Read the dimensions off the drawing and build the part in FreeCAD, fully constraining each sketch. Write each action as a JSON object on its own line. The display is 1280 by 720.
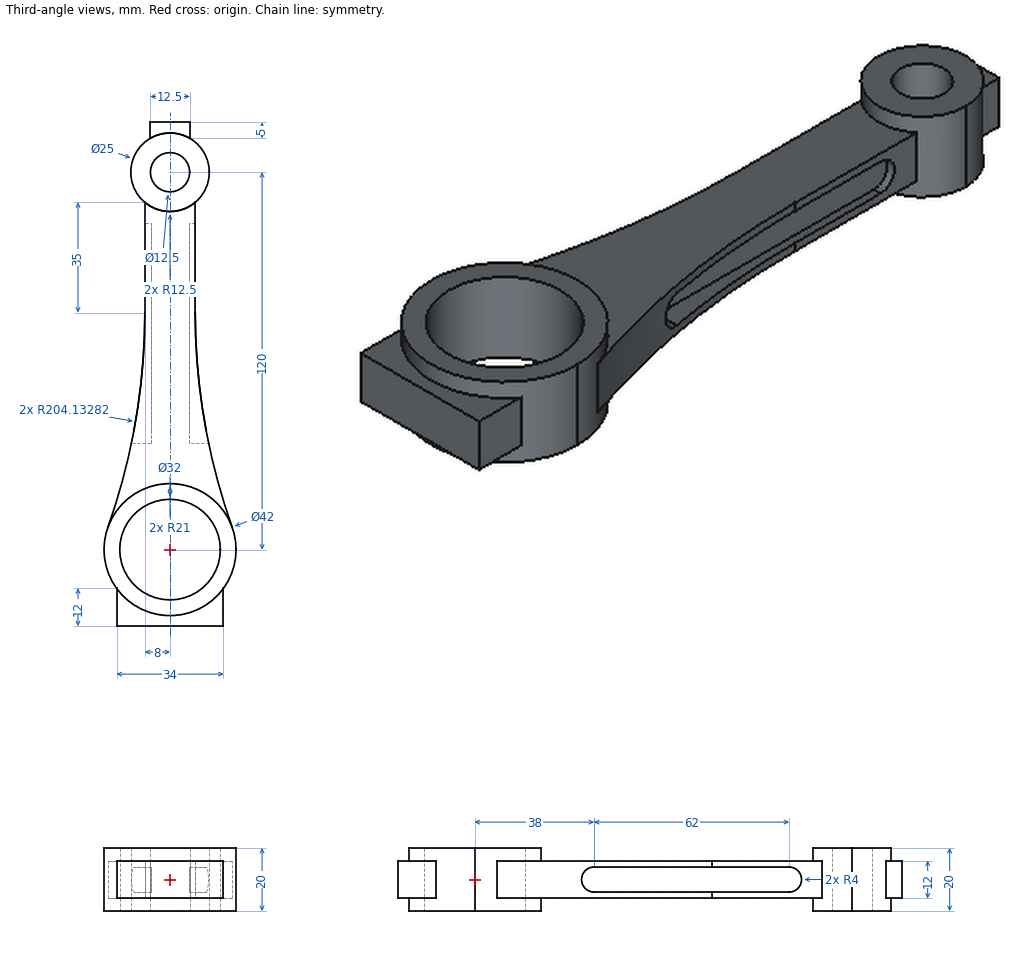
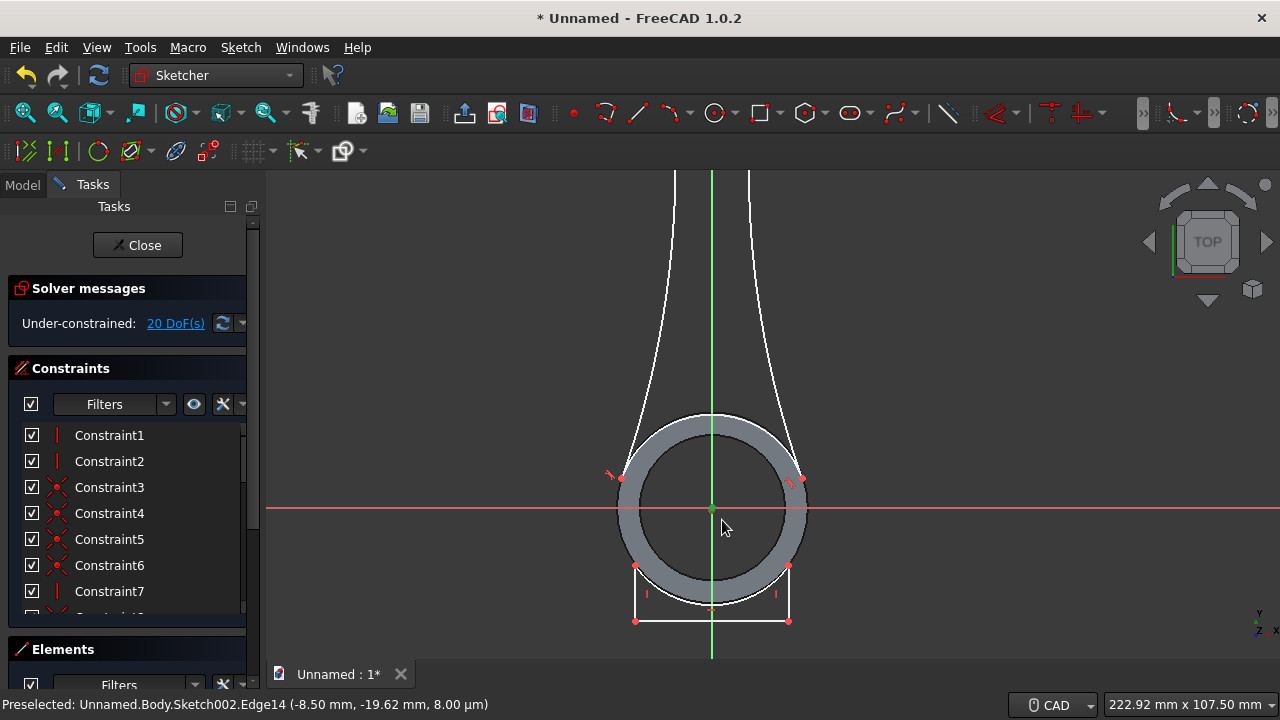
{"action": "key", "text": "c"}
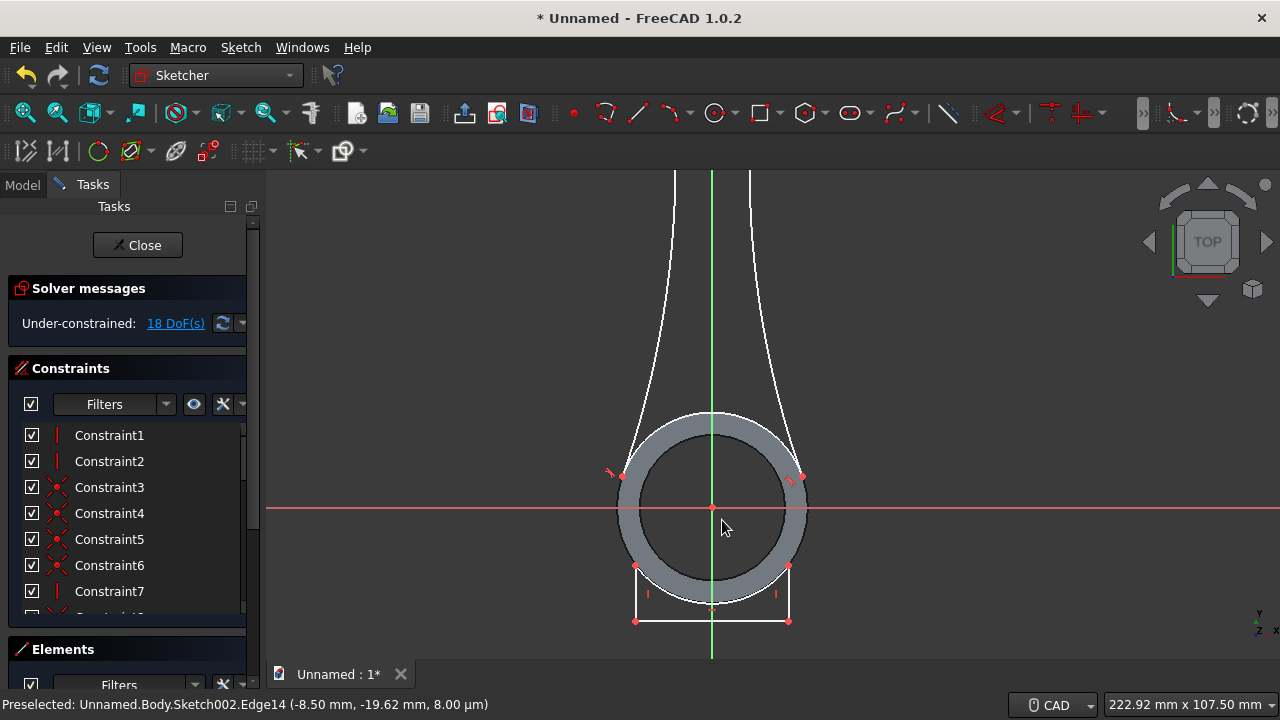
{"action": "left_click", "coordinate": [649, 386]}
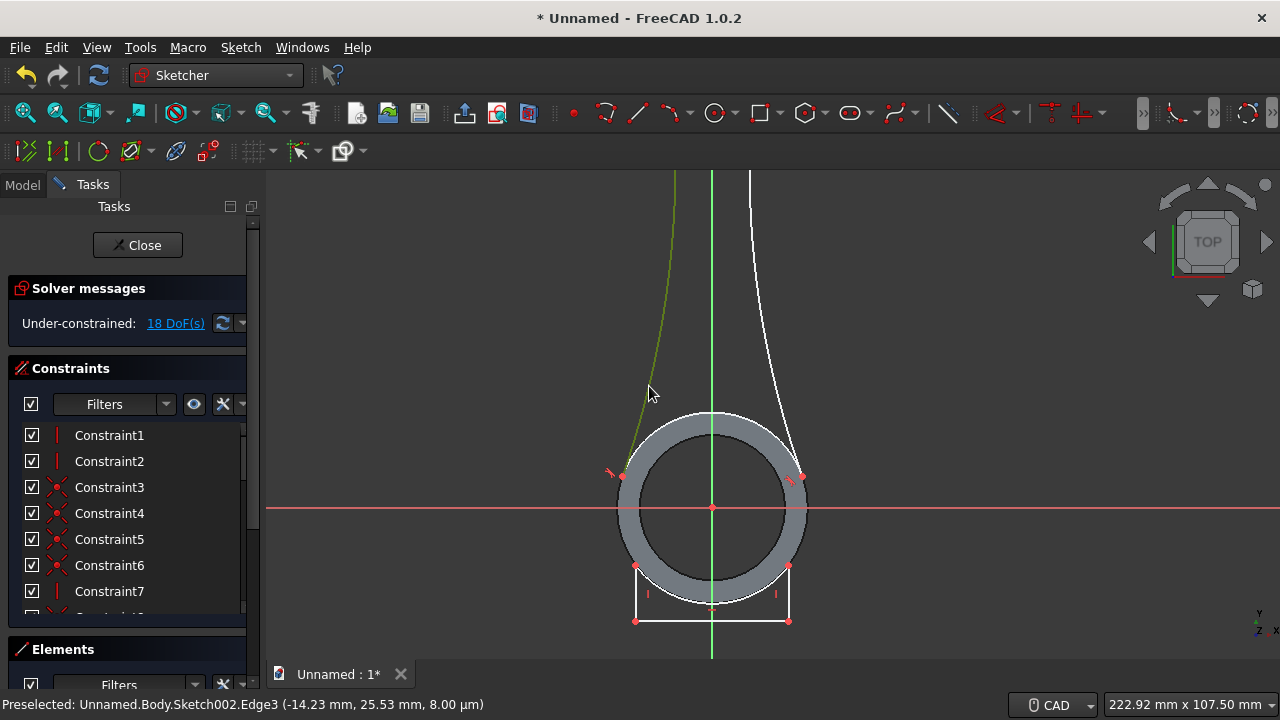
{"action": "left_click", "coordinate": [754, 261]}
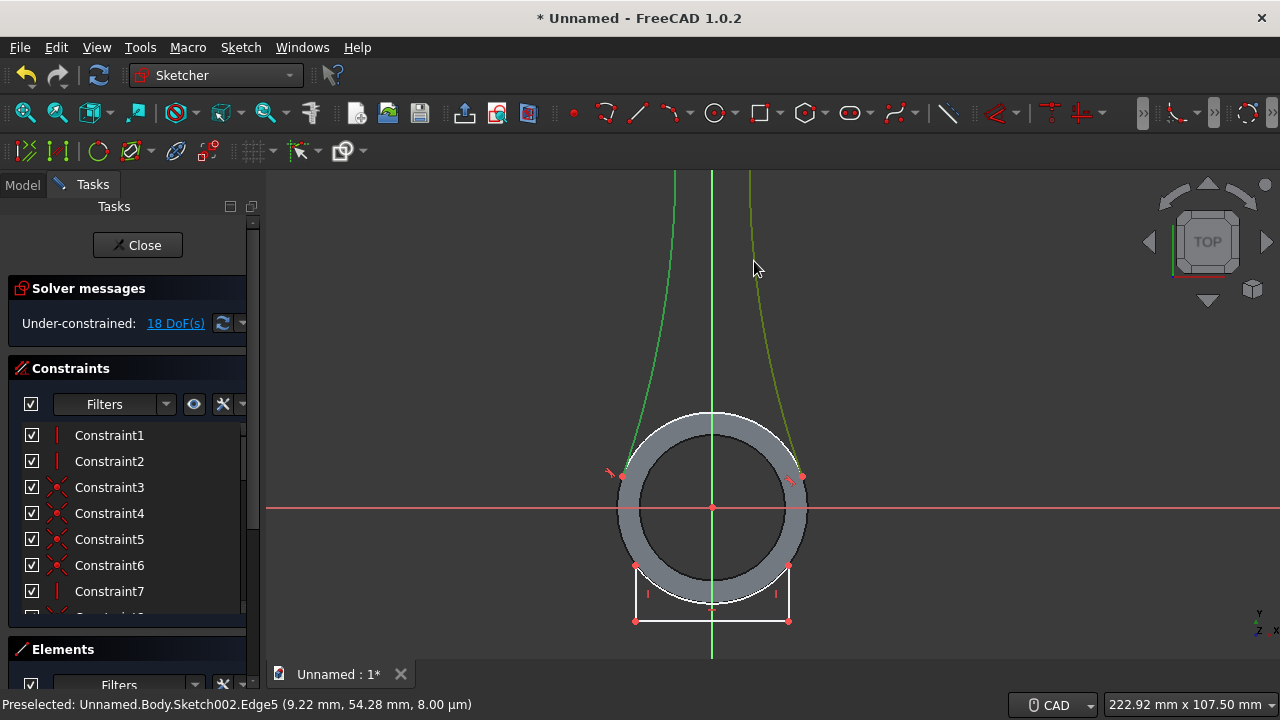
{"action": "key", "text": "e"}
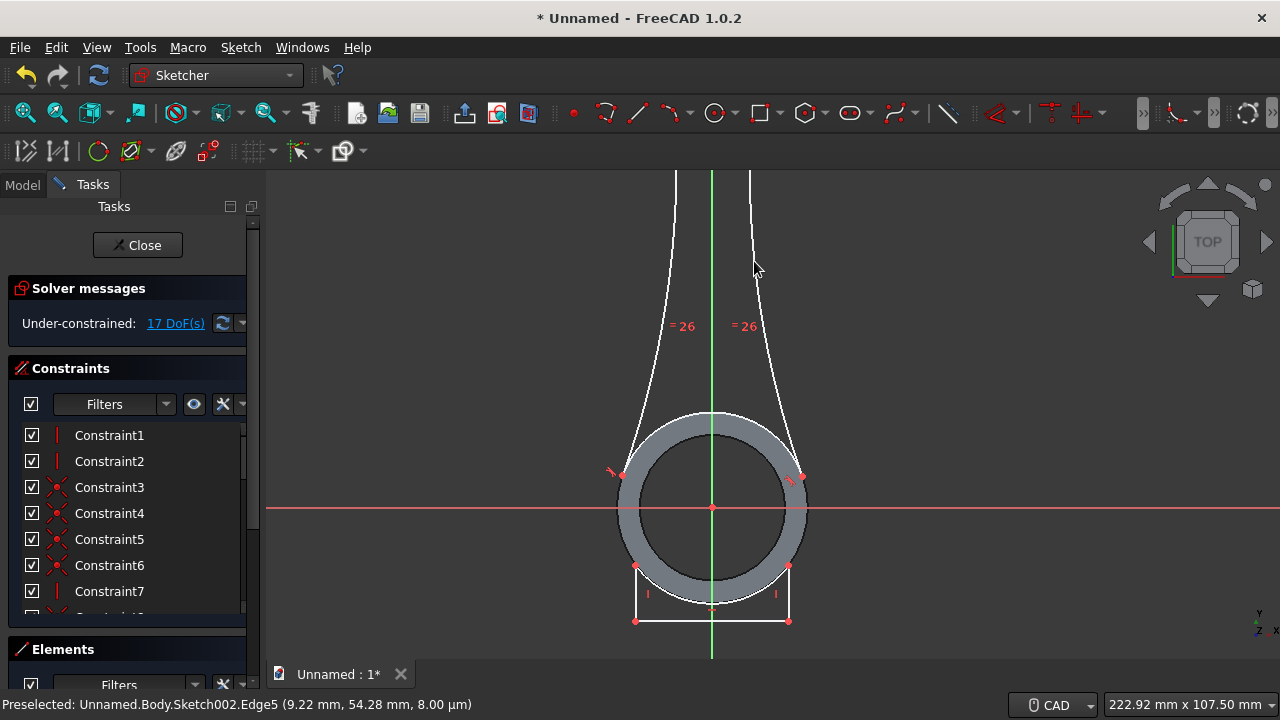
{"action": "scroll", "coordinate": [698, 545], "scroll_direction": "down", "scroll_amount": 4}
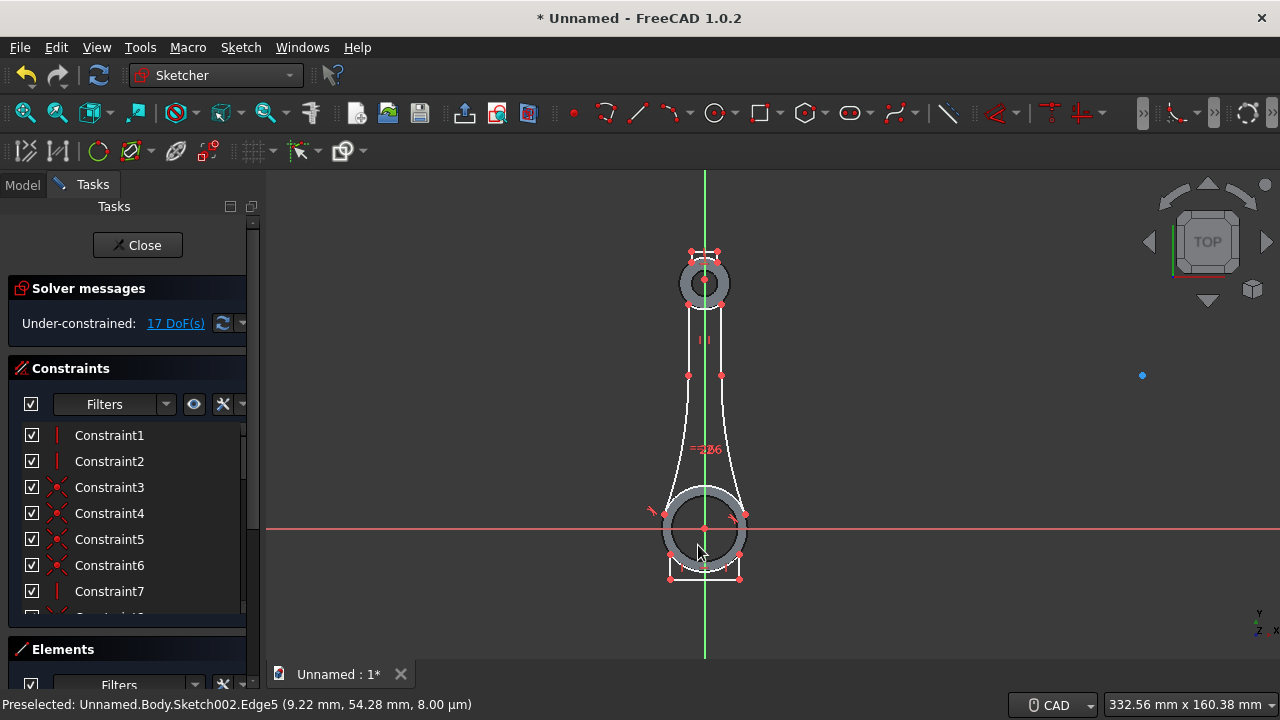
{"action": "scroll", "coordinate": [698, 309], "scroll_direction": "up", "scroll_amount": 4}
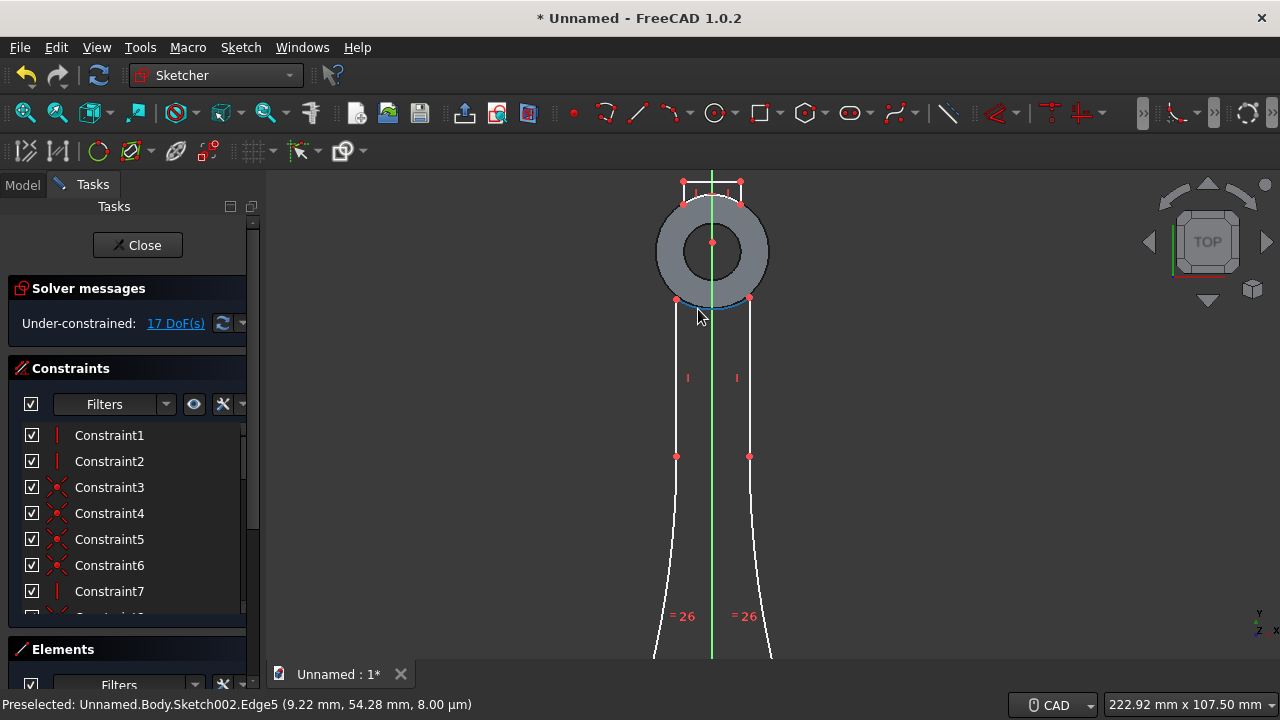
{"action": "left_click", "coordinate": [698, 308]}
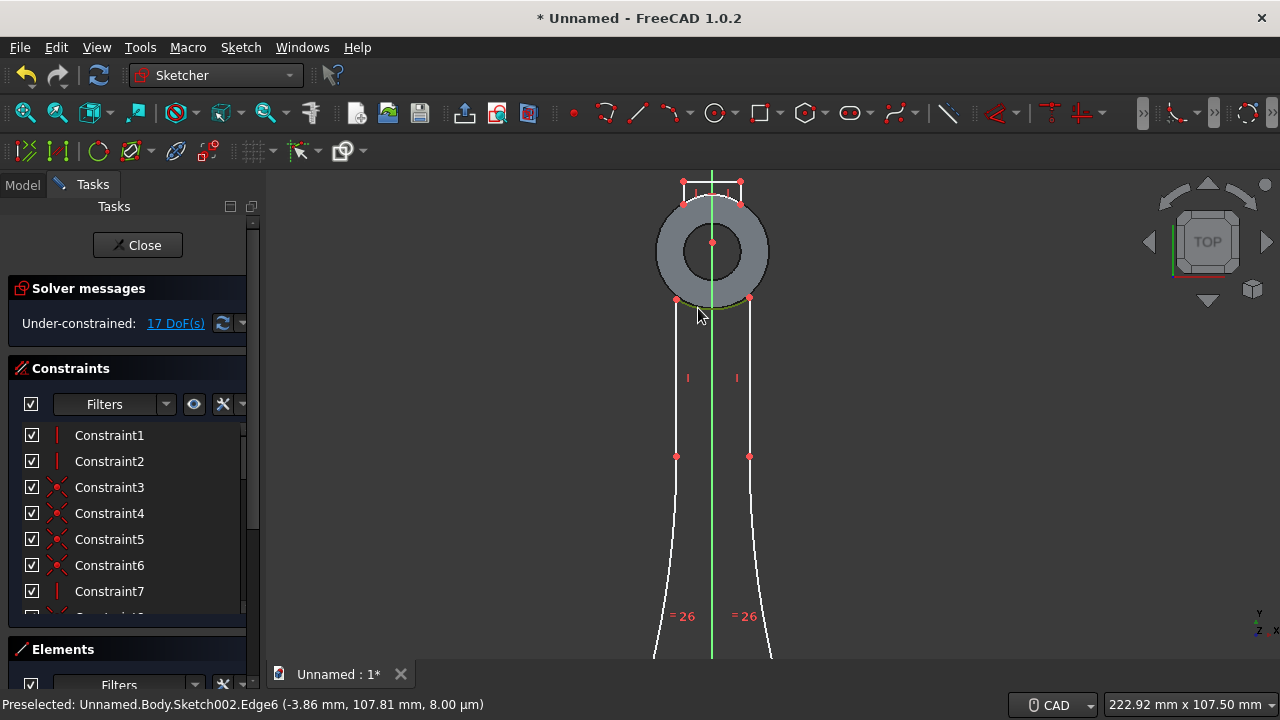
{"action": "scroll", "coordinate": [730, 198], "scroll_direction": "up", "scroll_amount": 2}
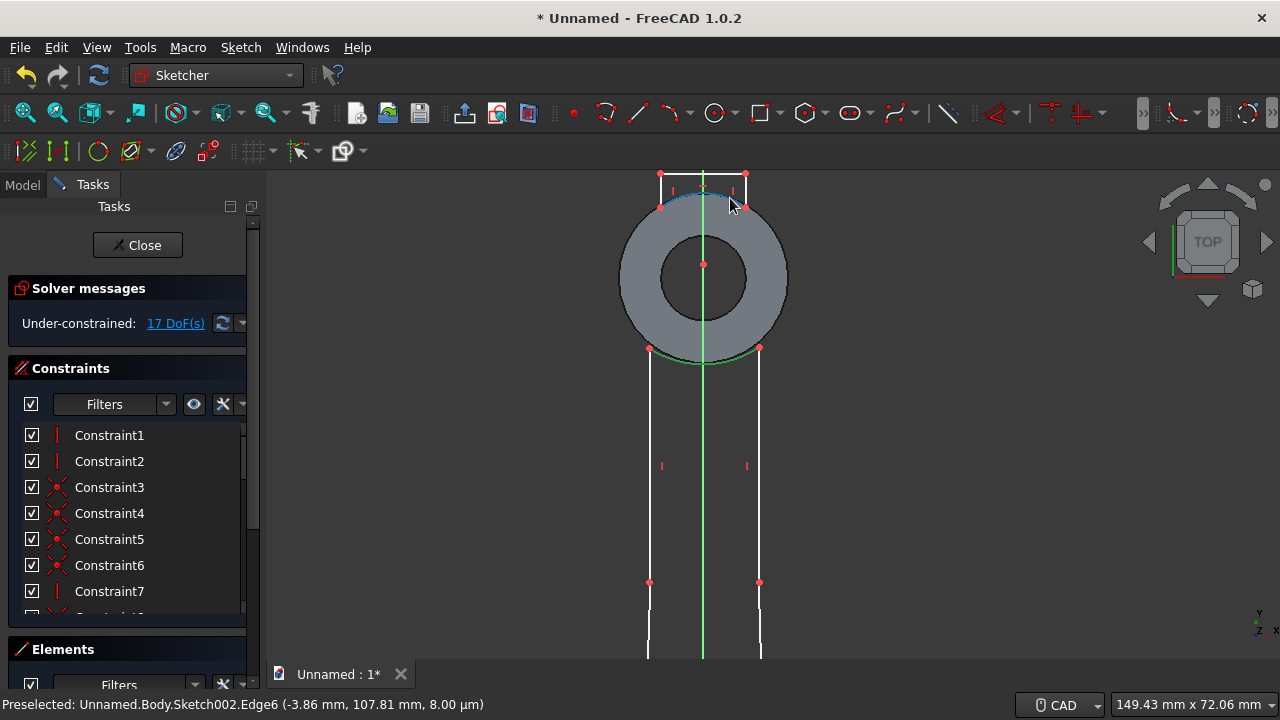
{"action": "left_click", "coordinate": [730, 198]}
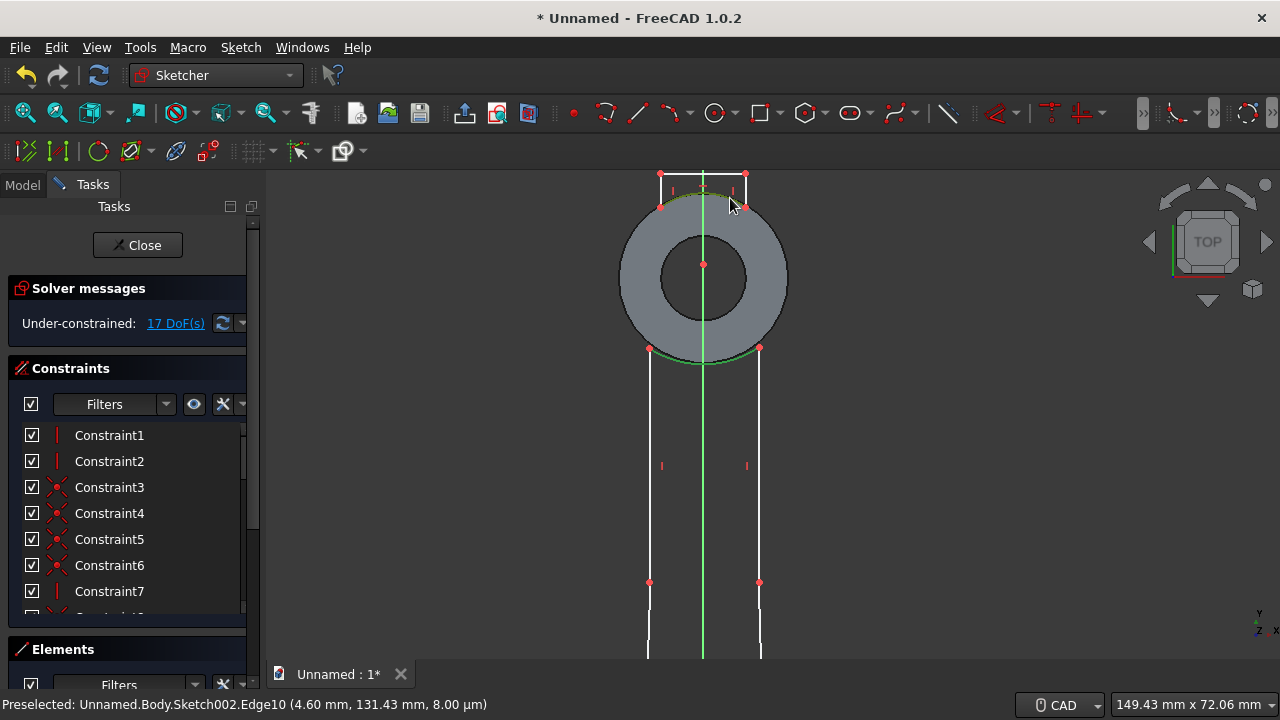
{"action": "key", "text": "e"}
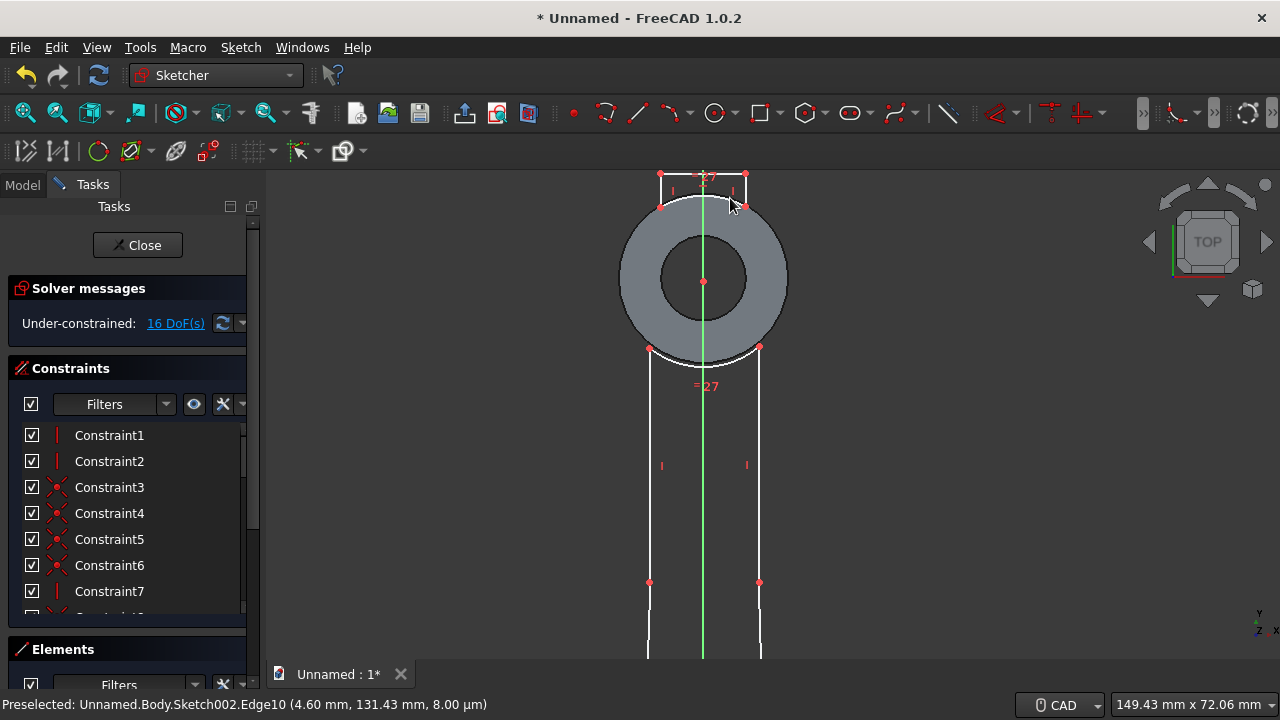
{"action": "scroll", "coordinate": [705, 285], "scroll_direction": "down", "scroll_amount": 6}